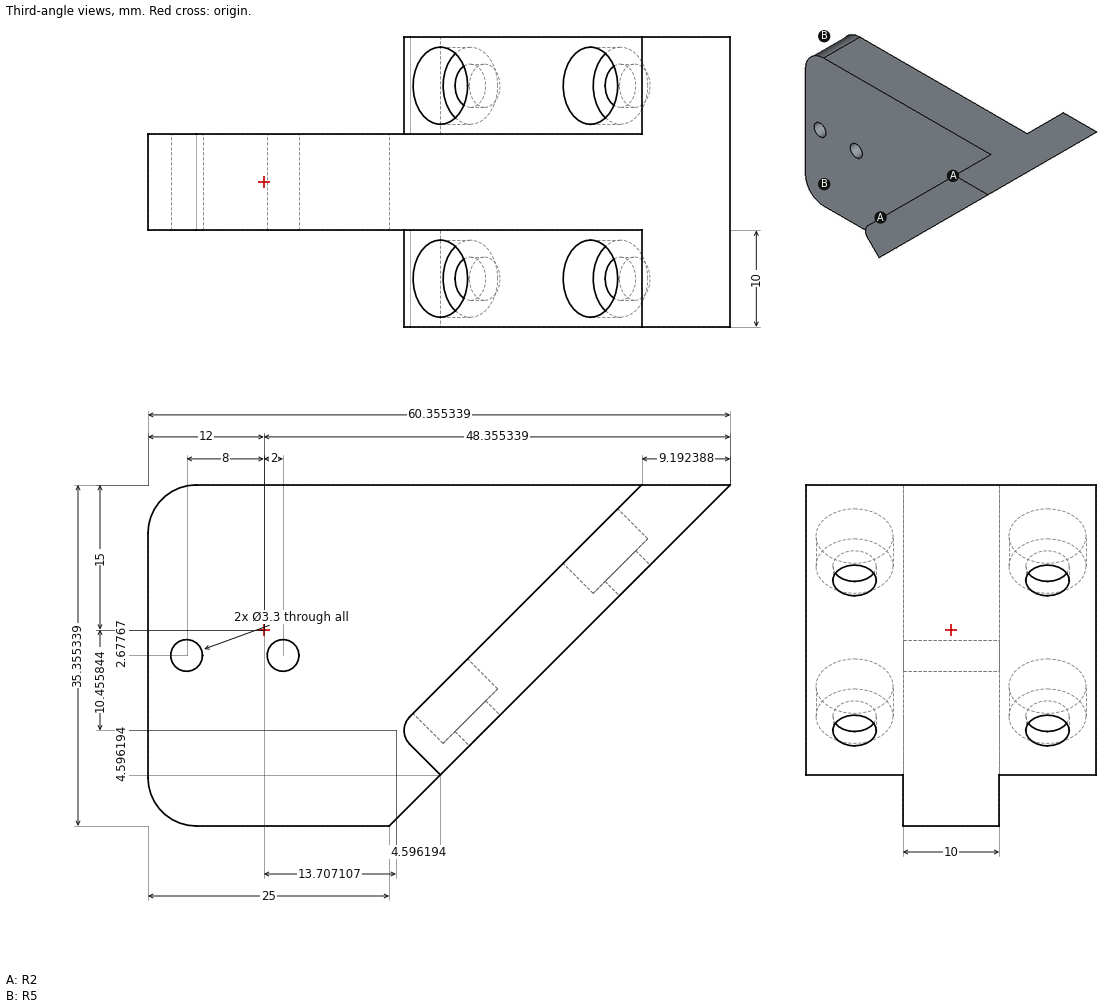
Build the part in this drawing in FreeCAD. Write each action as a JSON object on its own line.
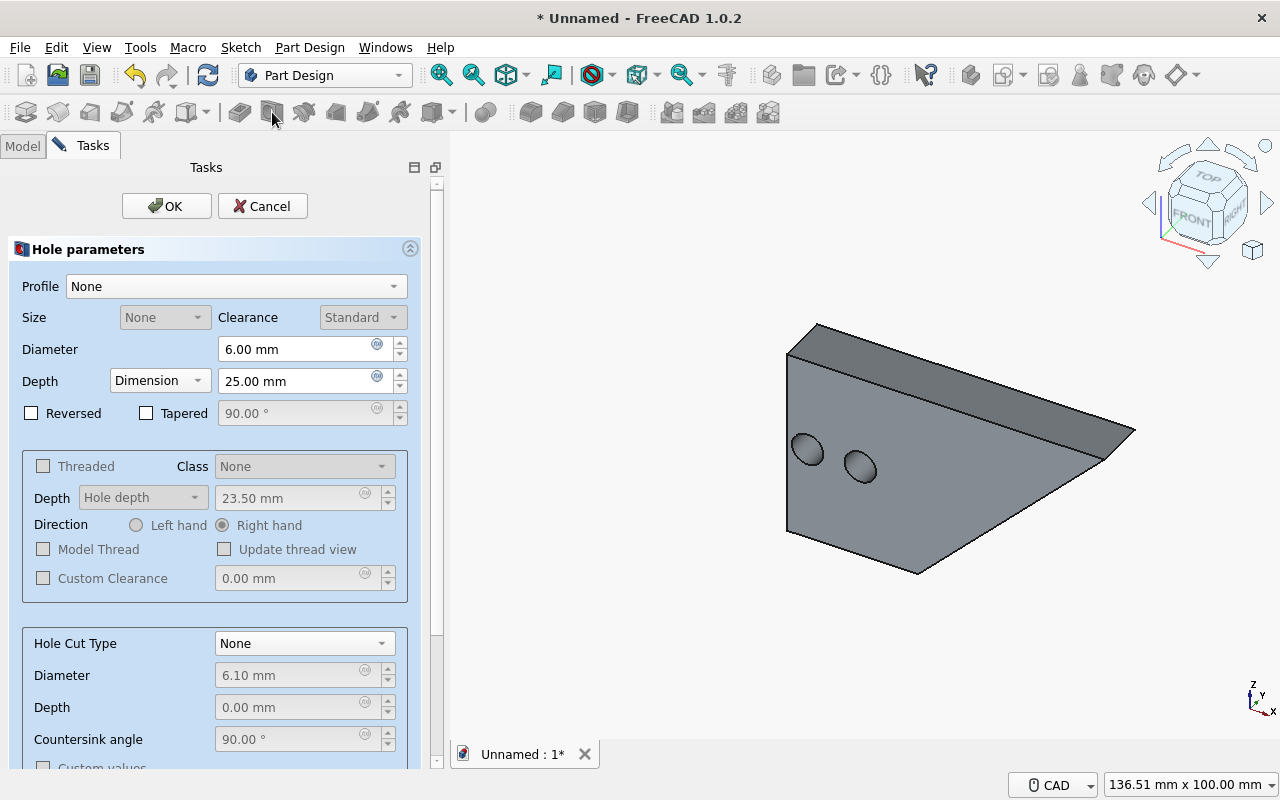
{"action": "triple_click", "coordinate": [305, 349]}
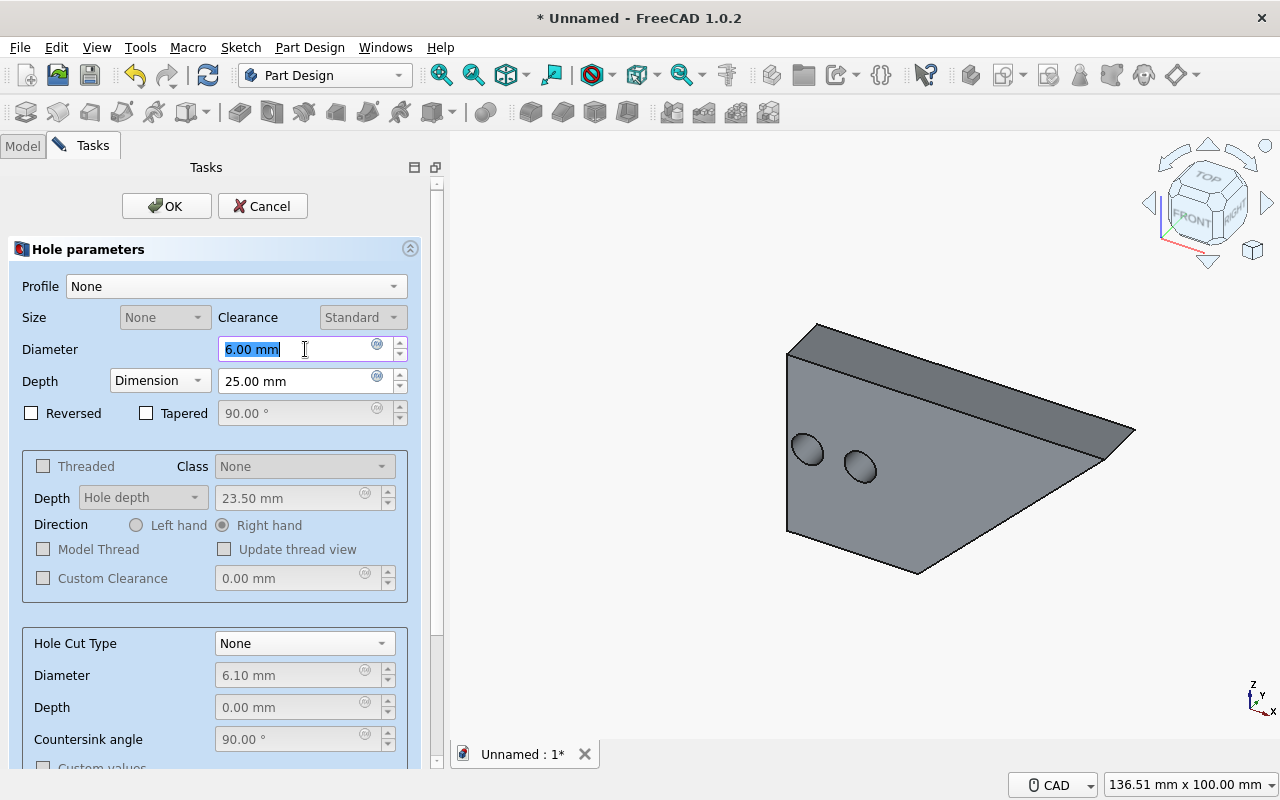
{"action": "type", "text": "3.3"}
{"action": "key", "text": "Tab"}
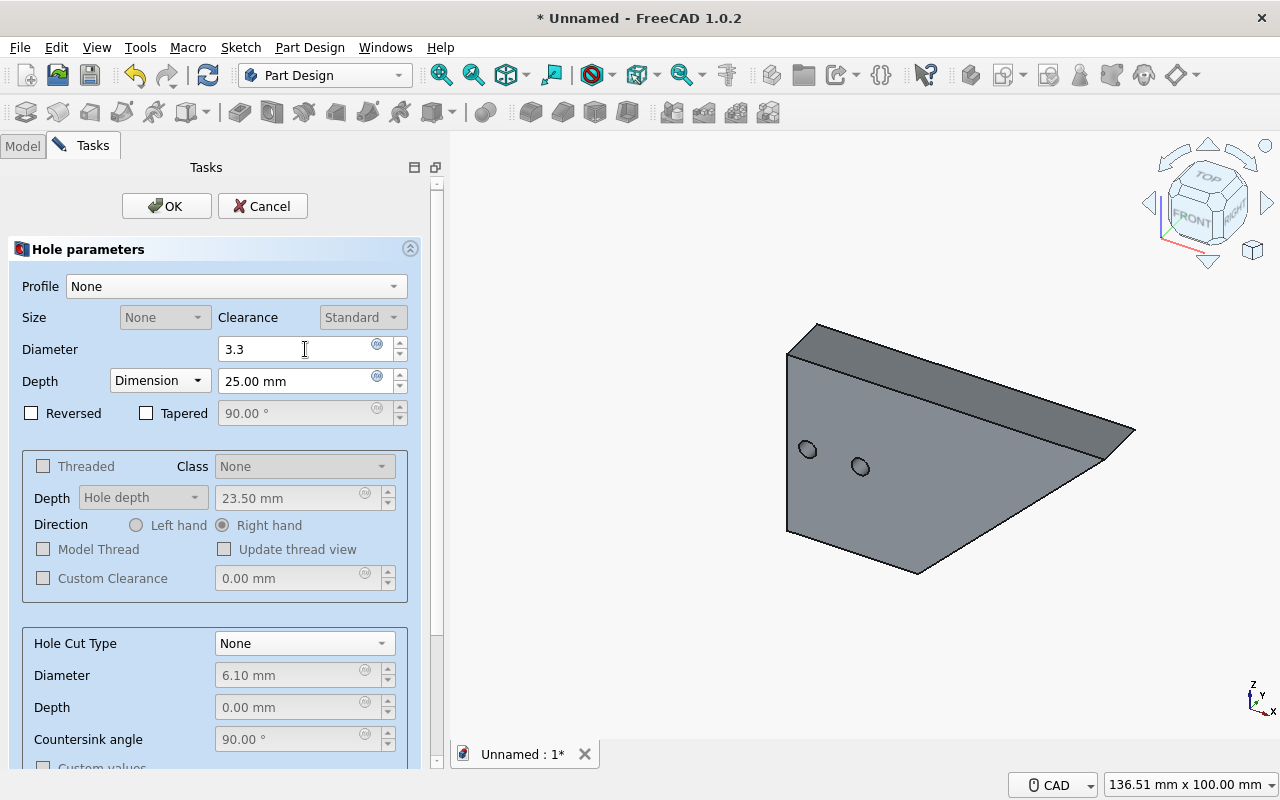
{"action": "left_click", "coordinate": [161, 380]}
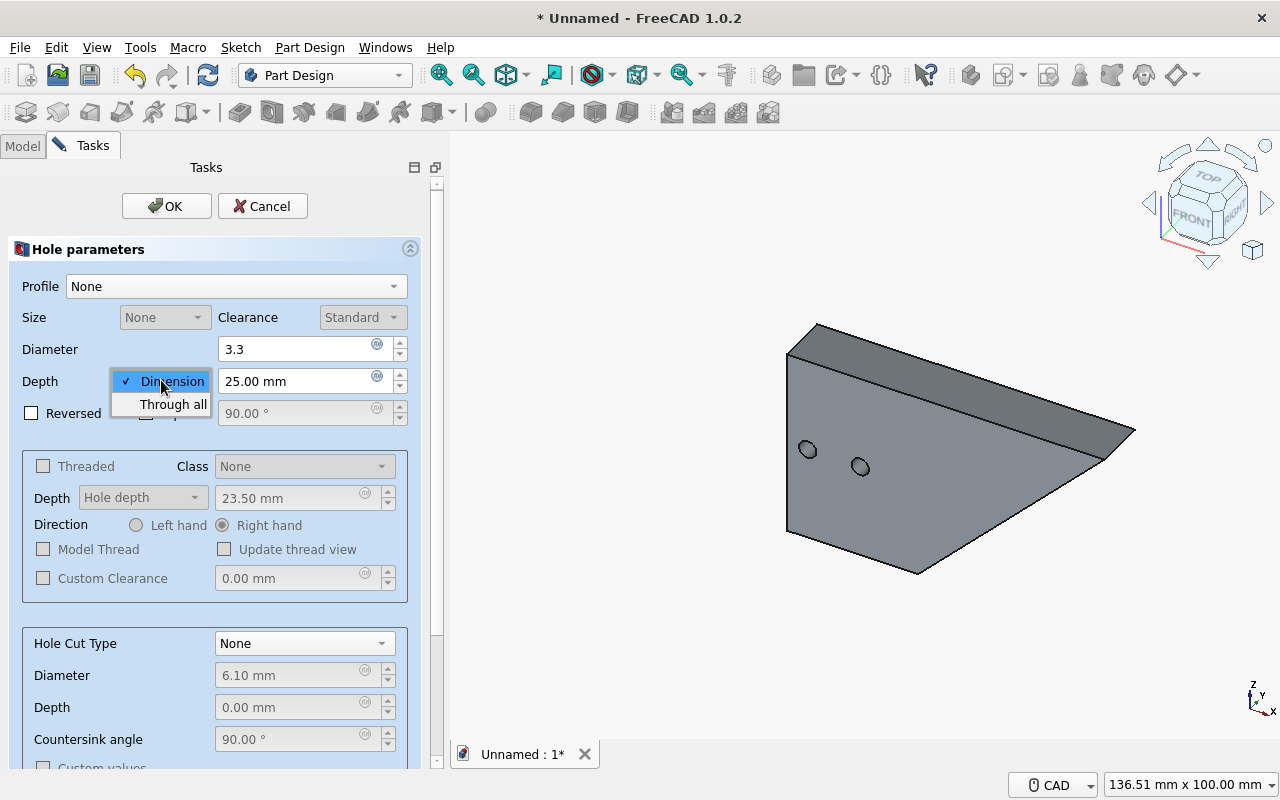
{"action": "left_click", "coordinate": [160, 404]}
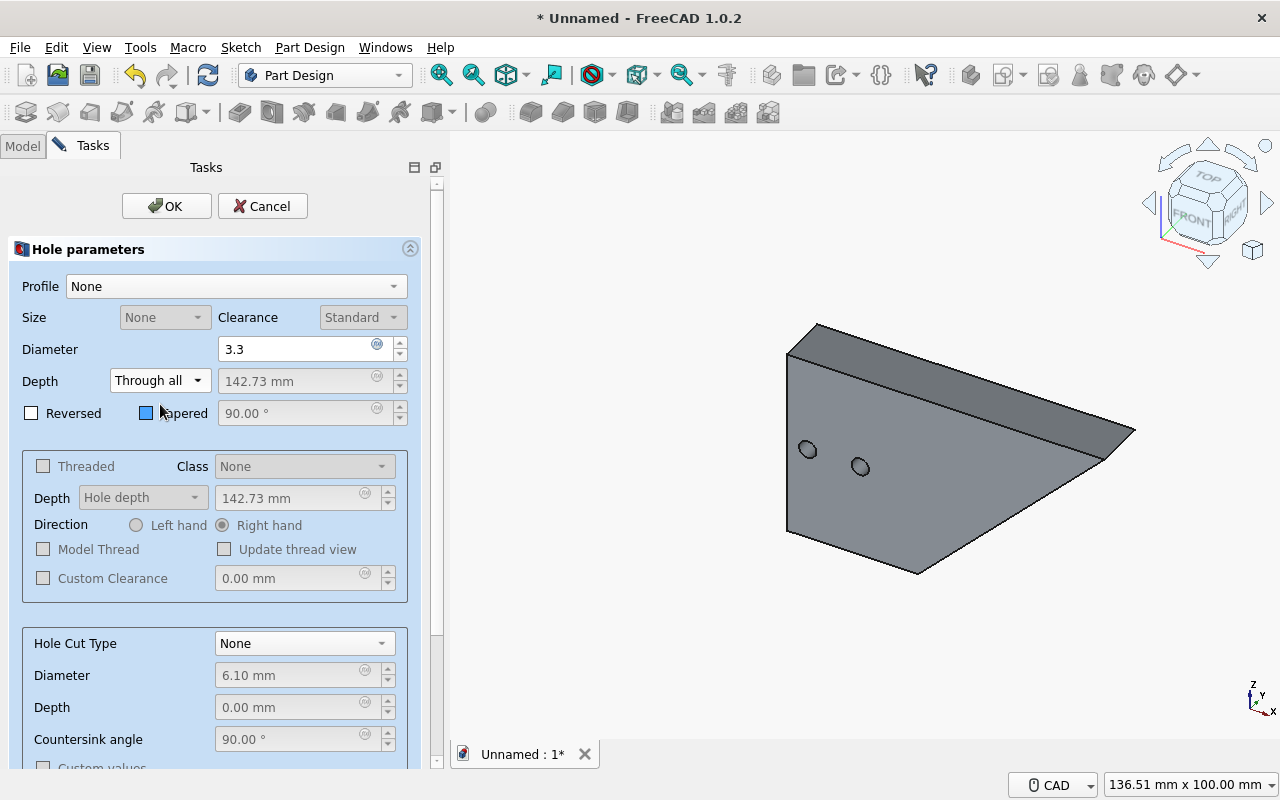
{"action": "left_click", "coordinate": [167, 206]}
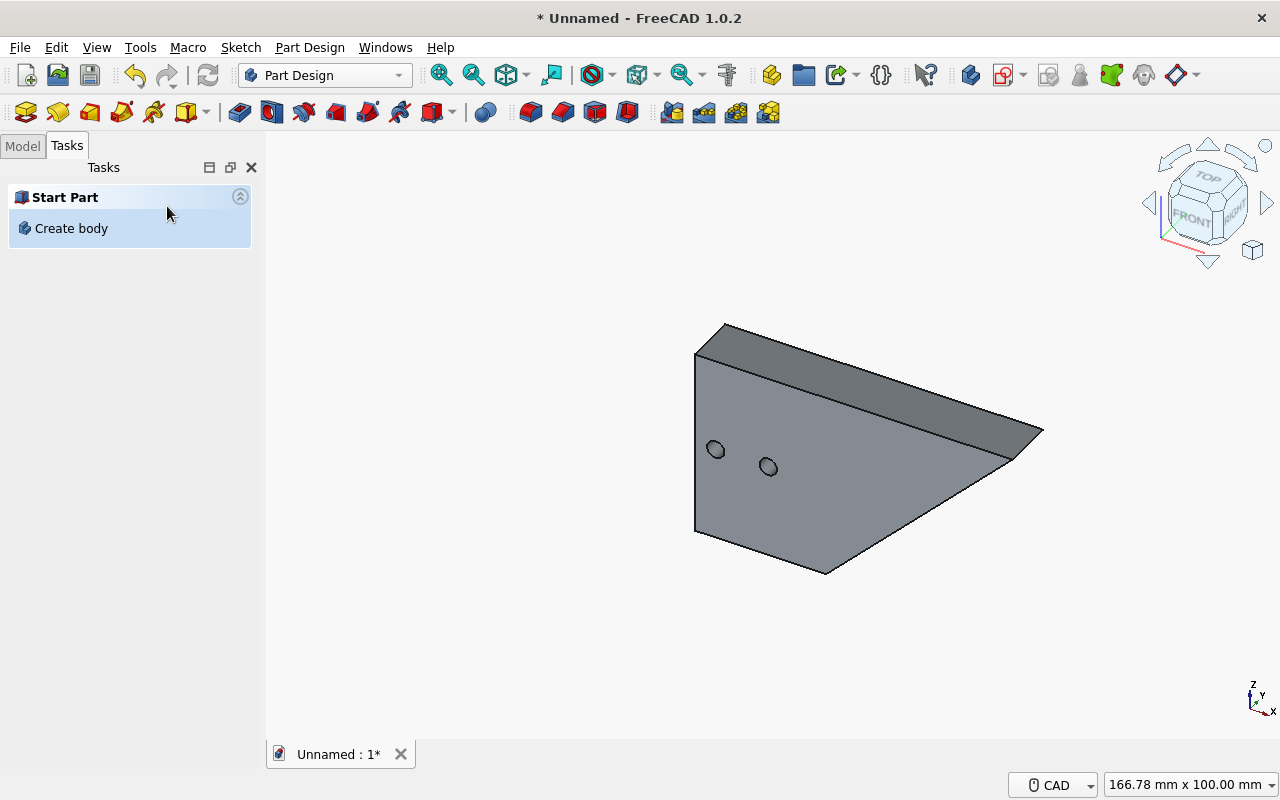
{"action": "left_click", "coordinate": [854, 469]}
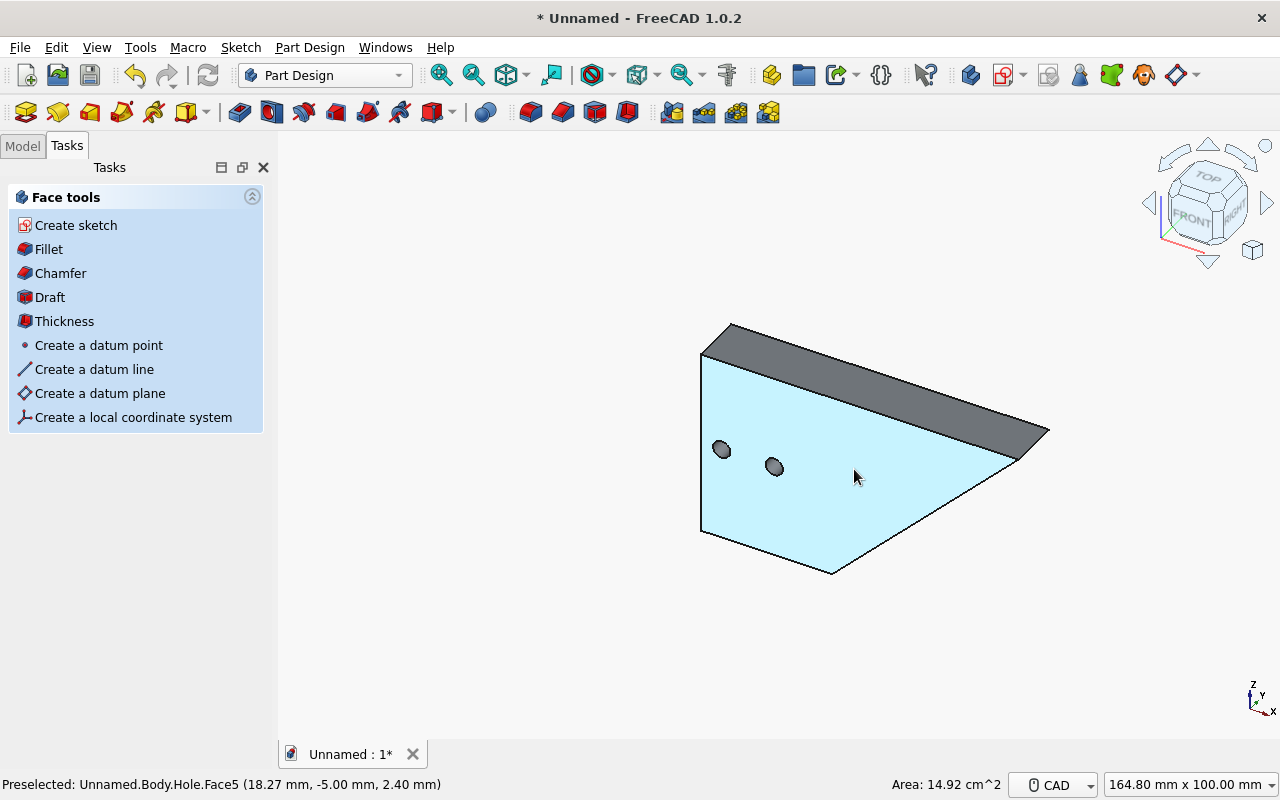
{"action": "left_click", "coordinate": [1004, 76]}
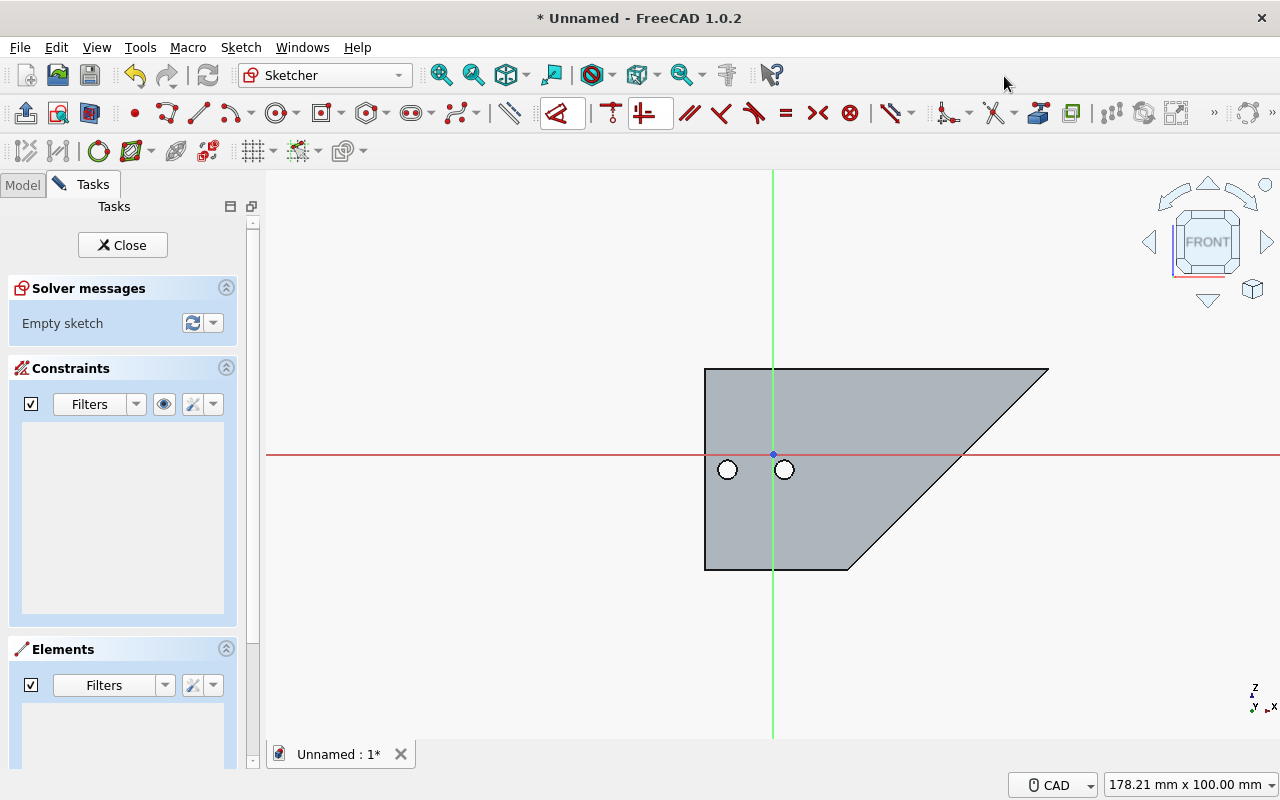
{"action": "scroll", "coordinate": [1079, 455], "scroll_direction": "up", "scroll_amount": 4}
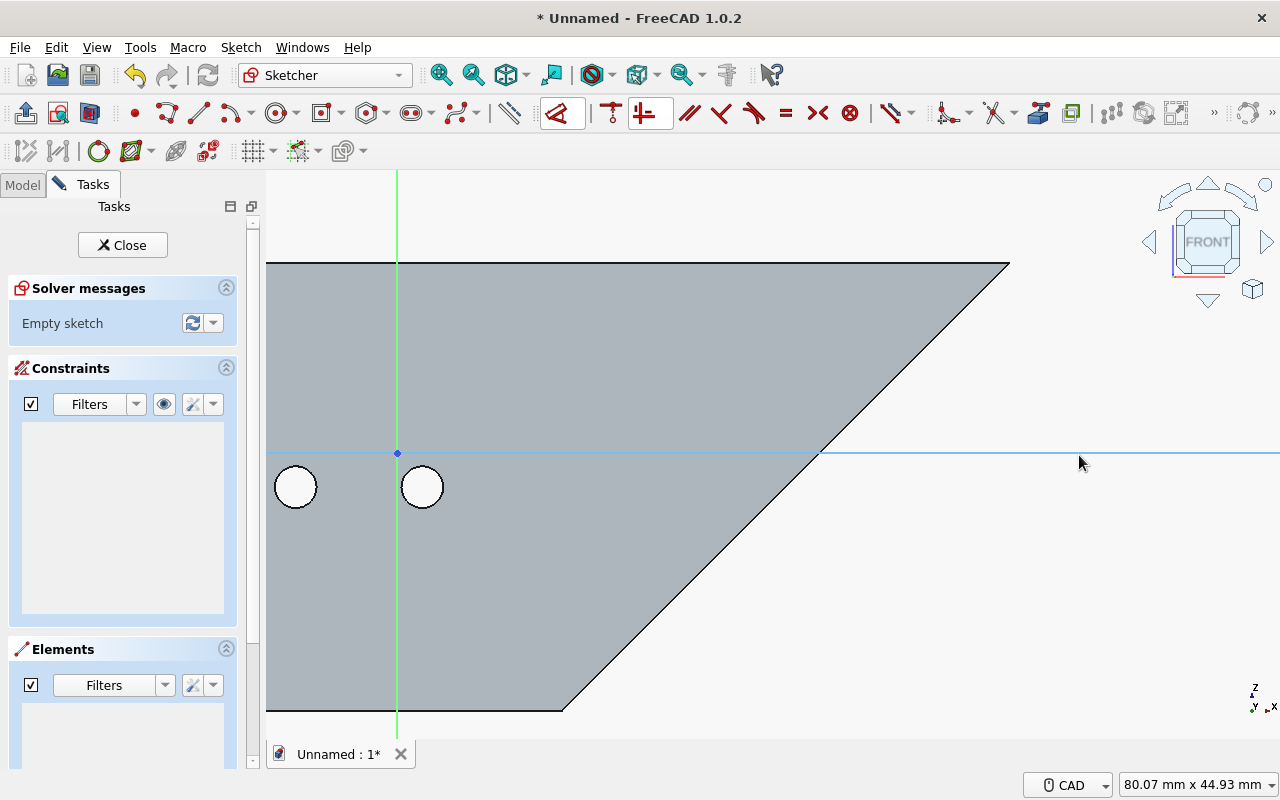
{"action": "left_click", "coordinate": [168, 114]}